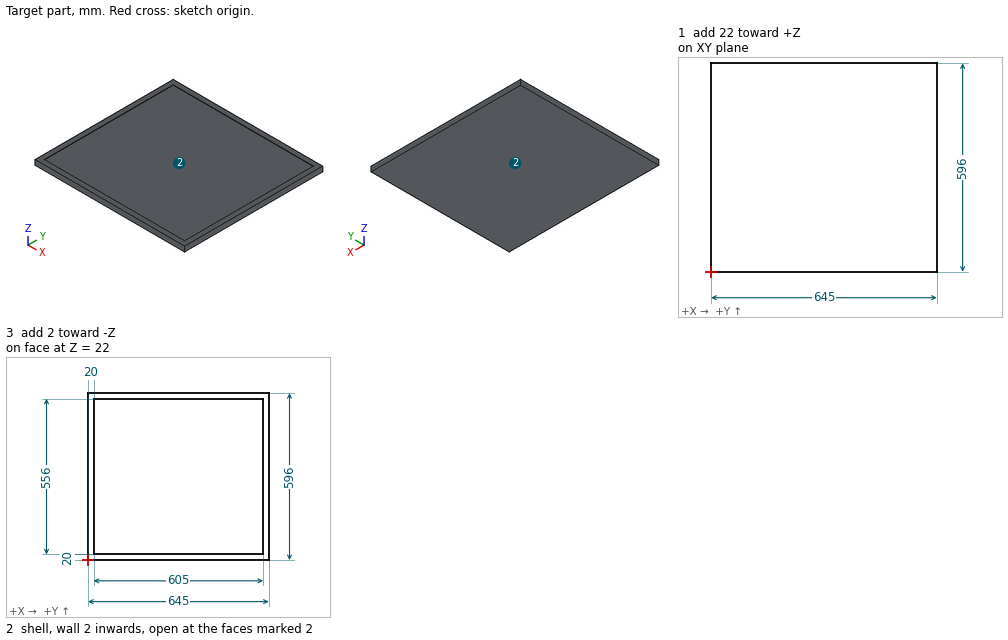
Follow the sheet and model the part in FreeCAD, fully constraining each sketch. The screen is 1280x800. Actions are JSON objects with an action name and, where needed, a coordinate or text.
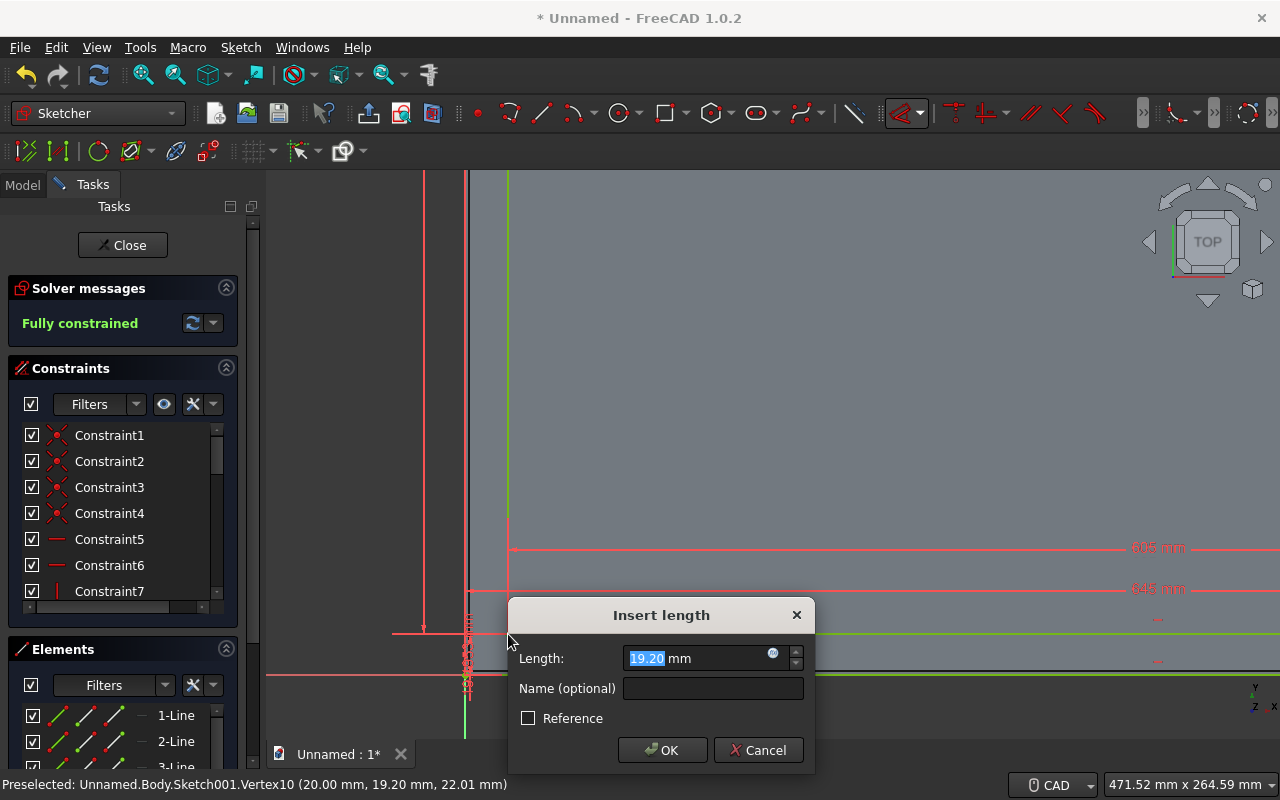
{"action": "type", "text": "20"}
{"action": "key", "text": "Return"}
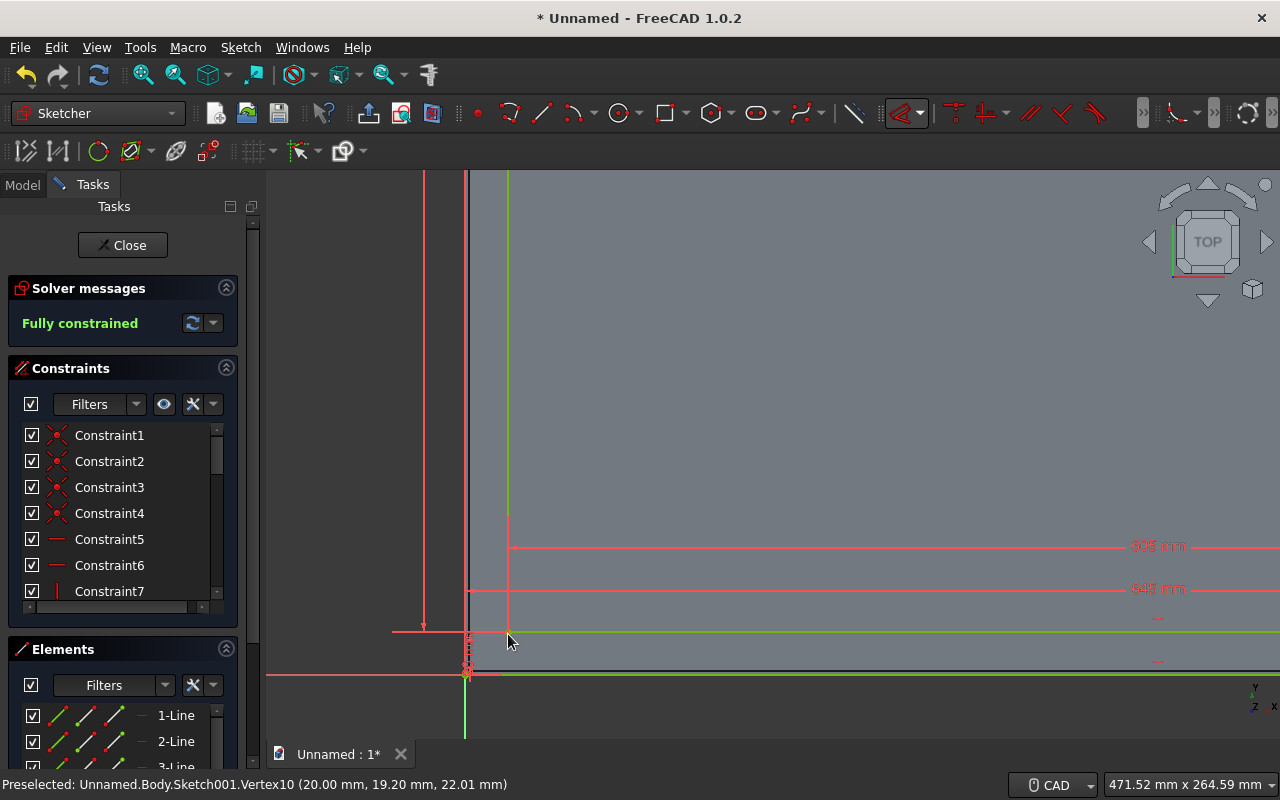
{"action": "left_click", "coordinate": [123, 245]}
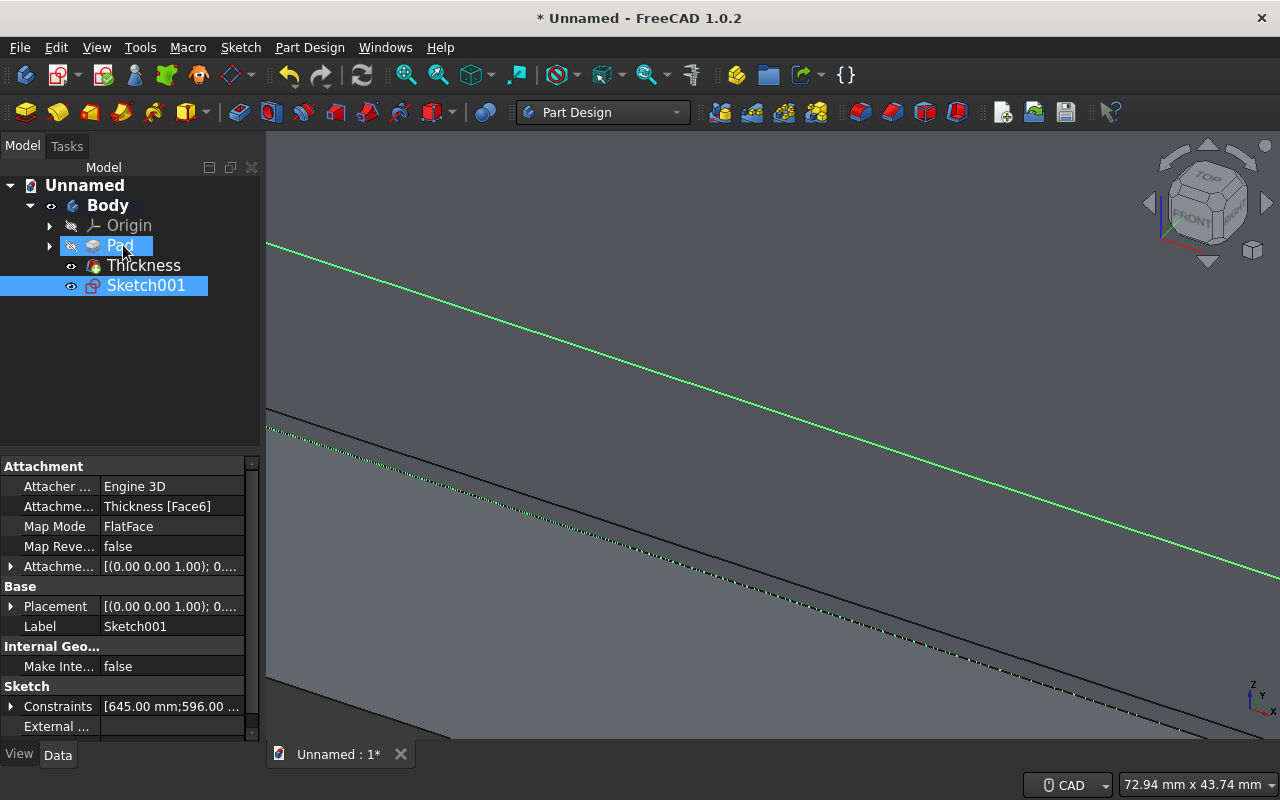
{"action": "left_click", "coordinate": [26, 112]}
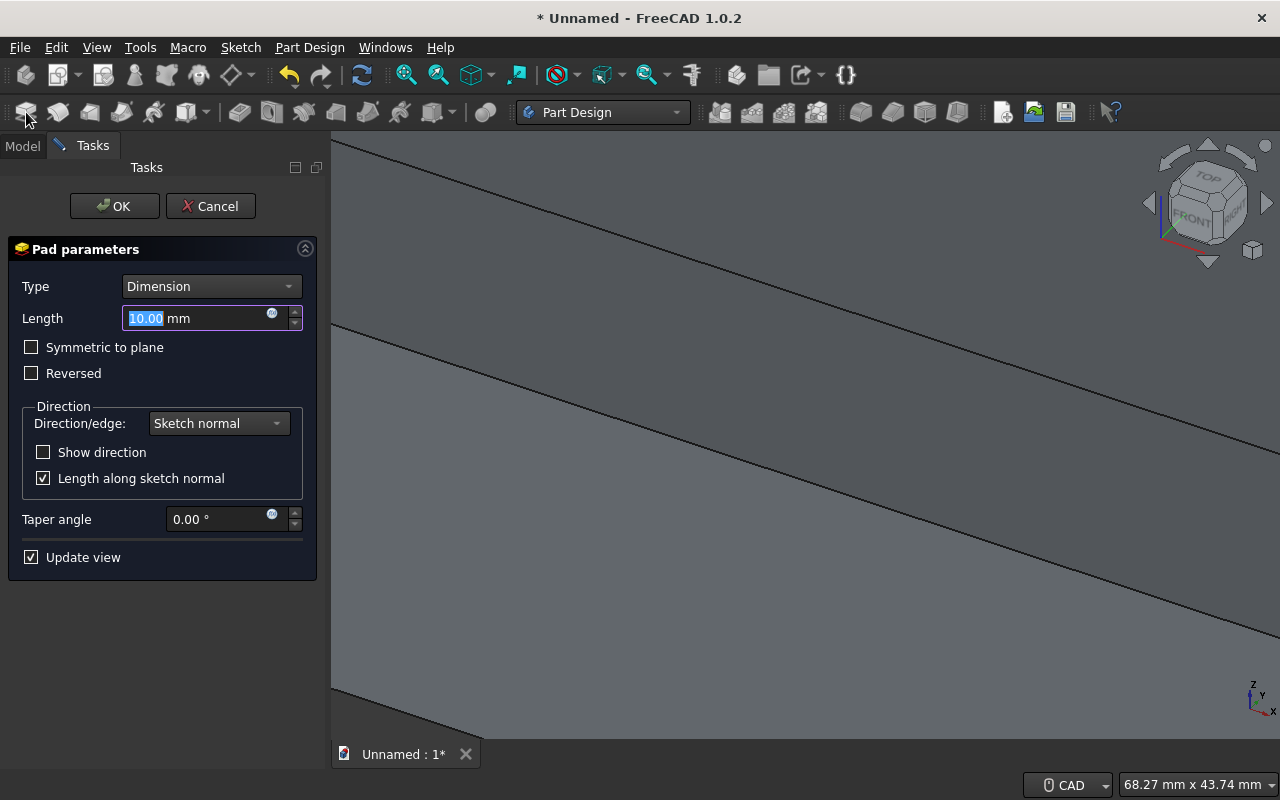
{"action": "type", "text": "2"}
{"action": "key", "text": "Tab"}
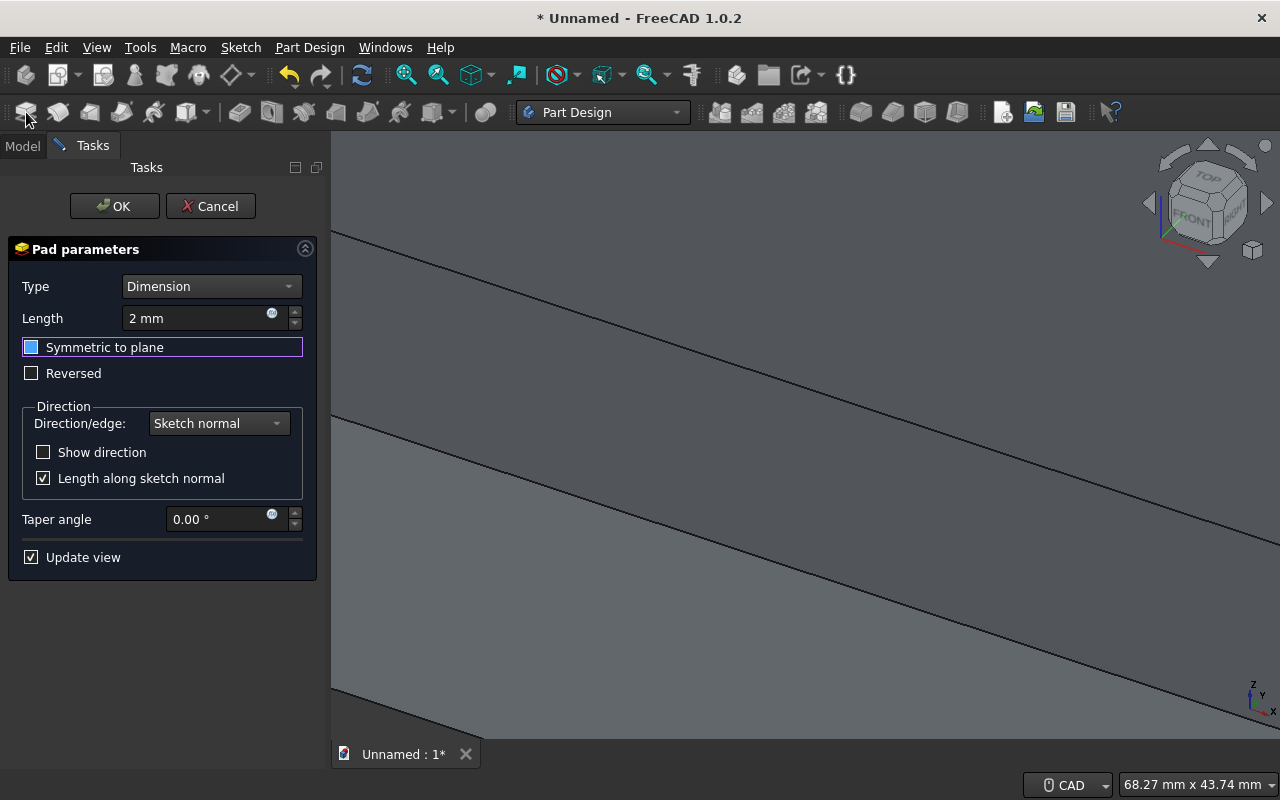
{"action": "left_click", "coordinate": [30, 373]}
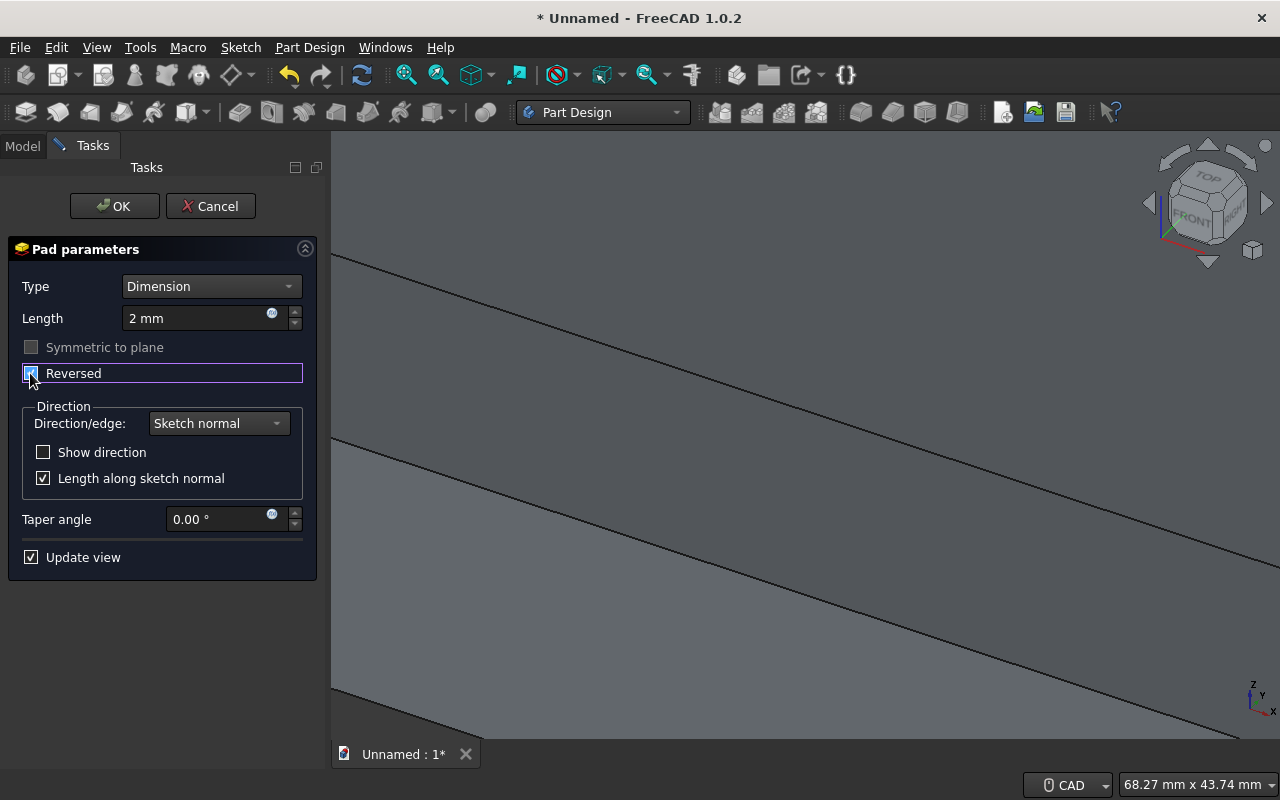
{"action": "left_click", "coordinate": [115, 206]}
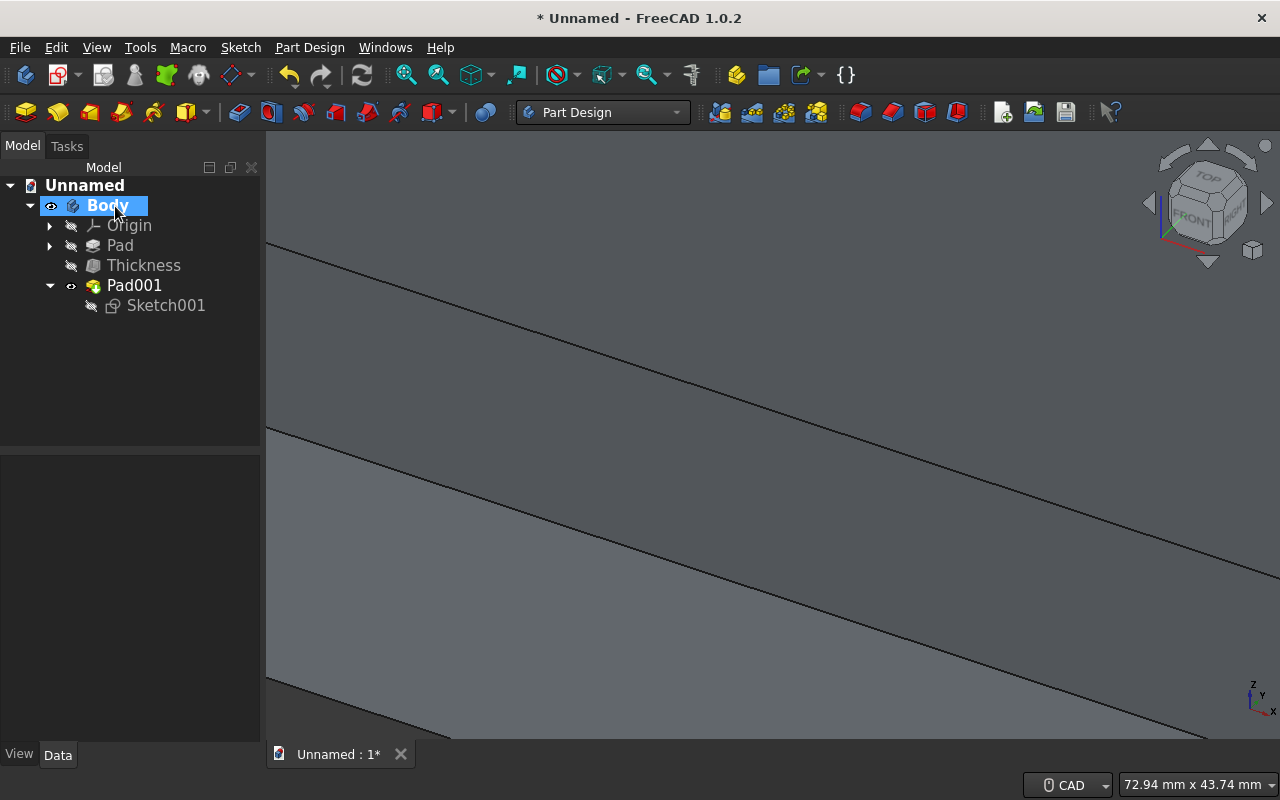
{"action": "key", "text": "0"}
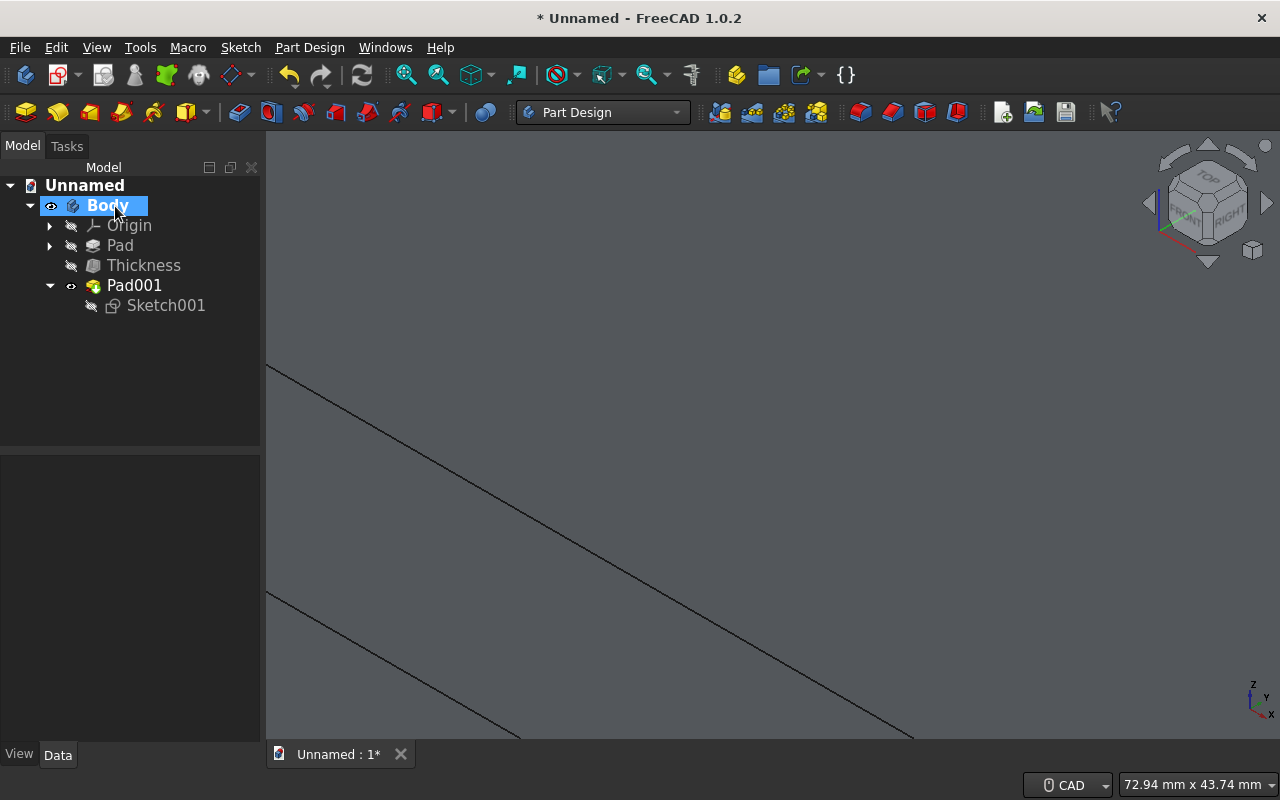
{"action": "left_click", "coordinate": [408, 76]}